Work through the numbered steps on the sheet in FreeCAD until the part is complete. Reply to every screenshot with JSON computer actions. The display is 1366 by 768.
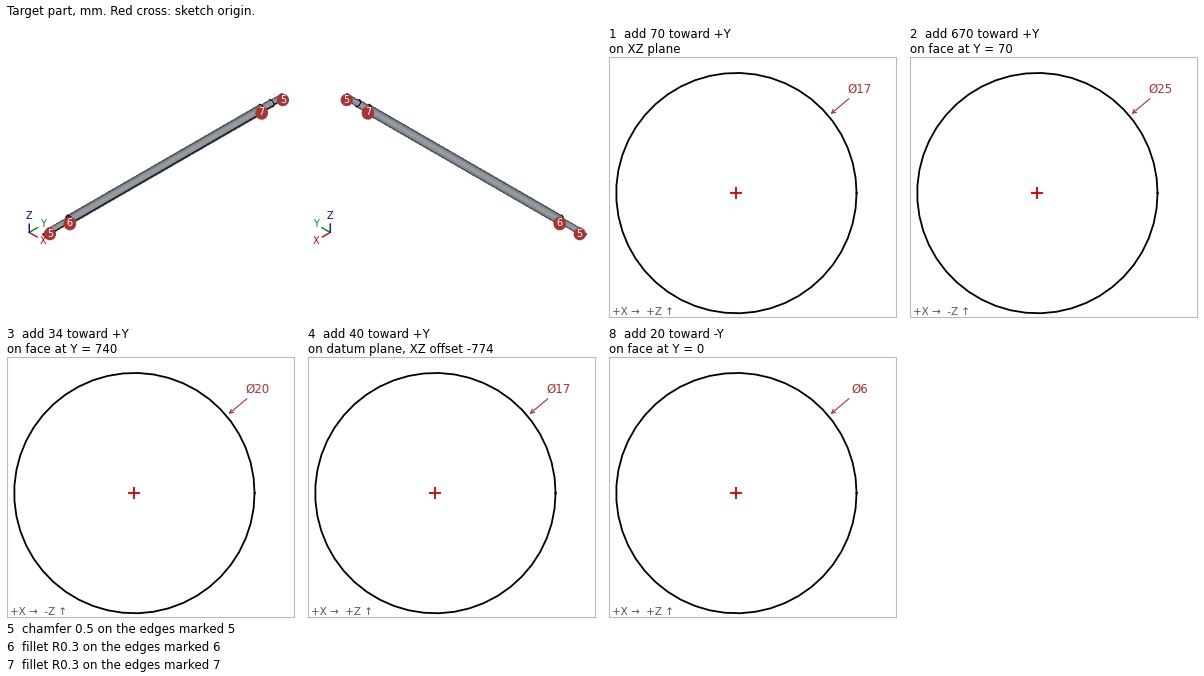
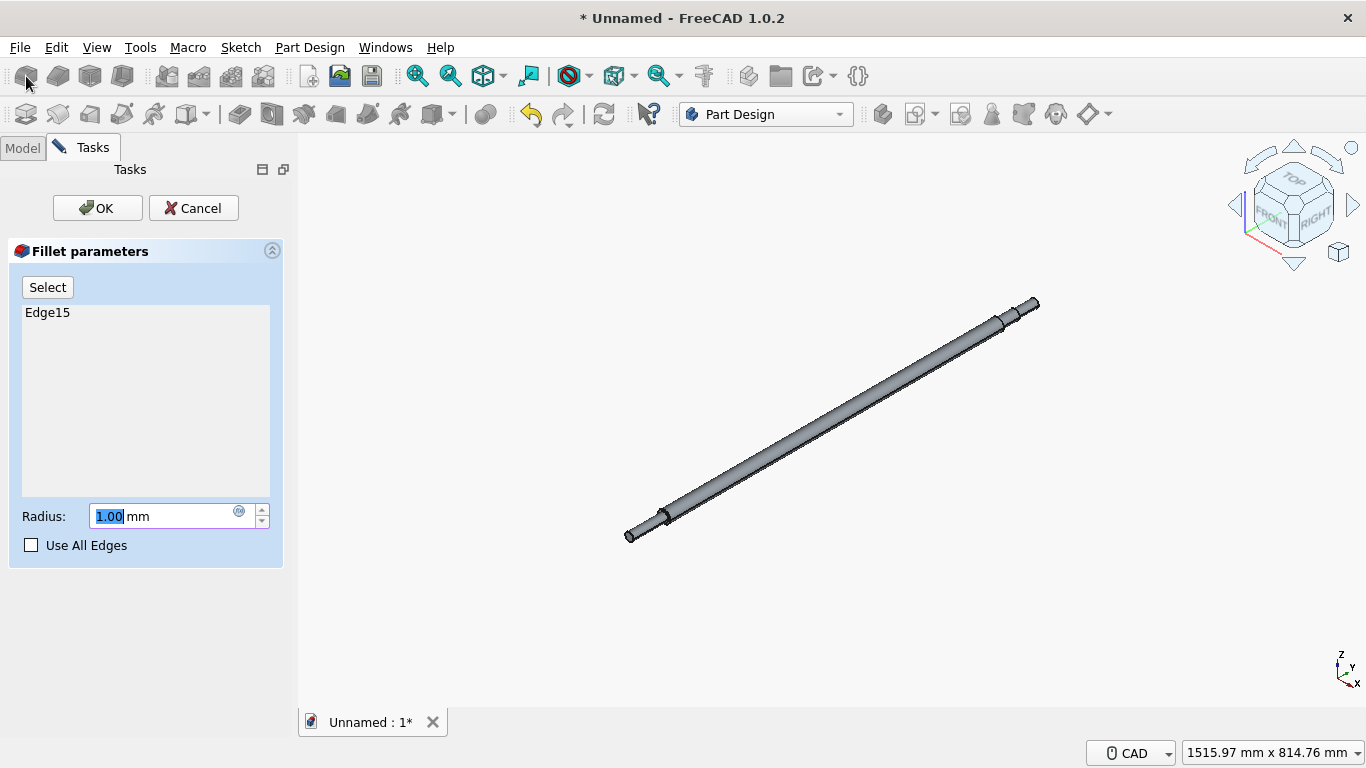
{"action": "type", "text": "0.3"}
{"action": "key", "text": "Tab"}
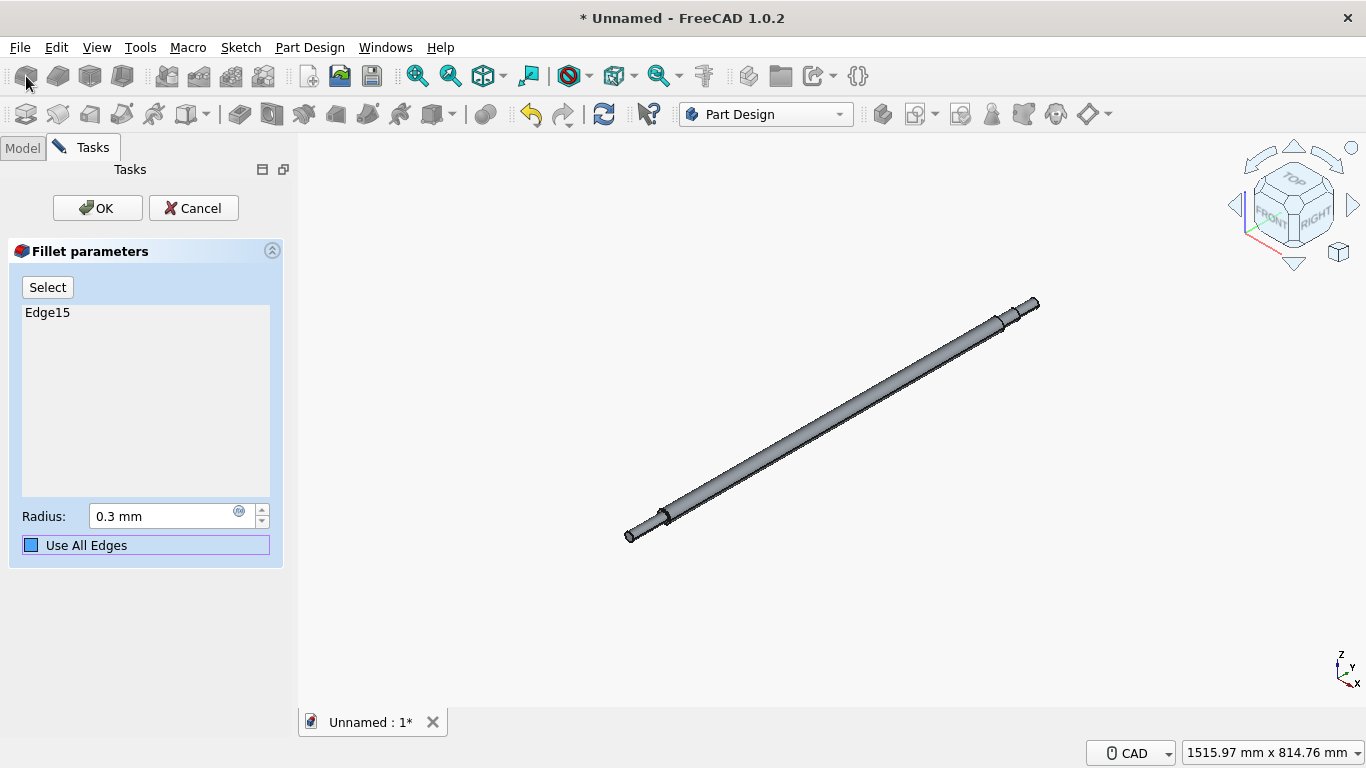
{"action": "left_click", "coordinate": [98, 208]}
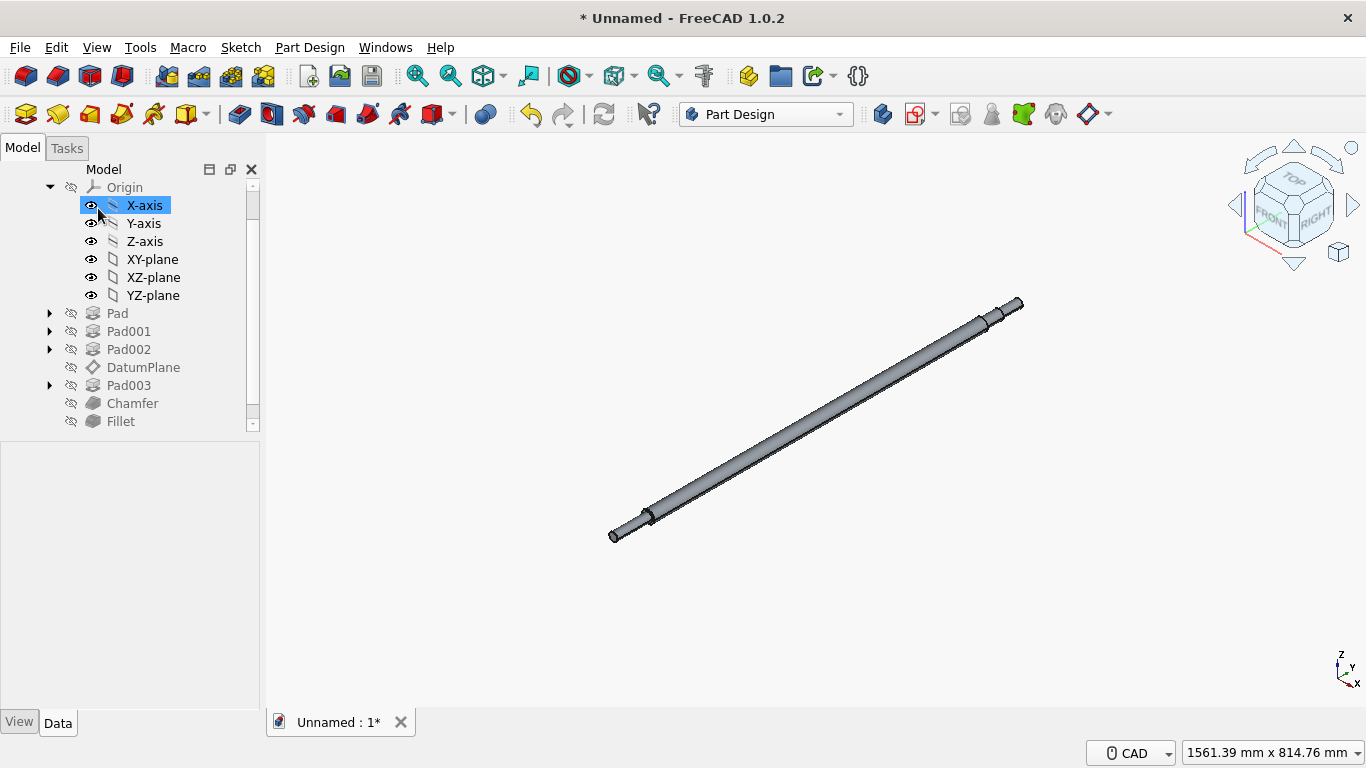
{"action": "left_click", "coordinate": [418, 76]}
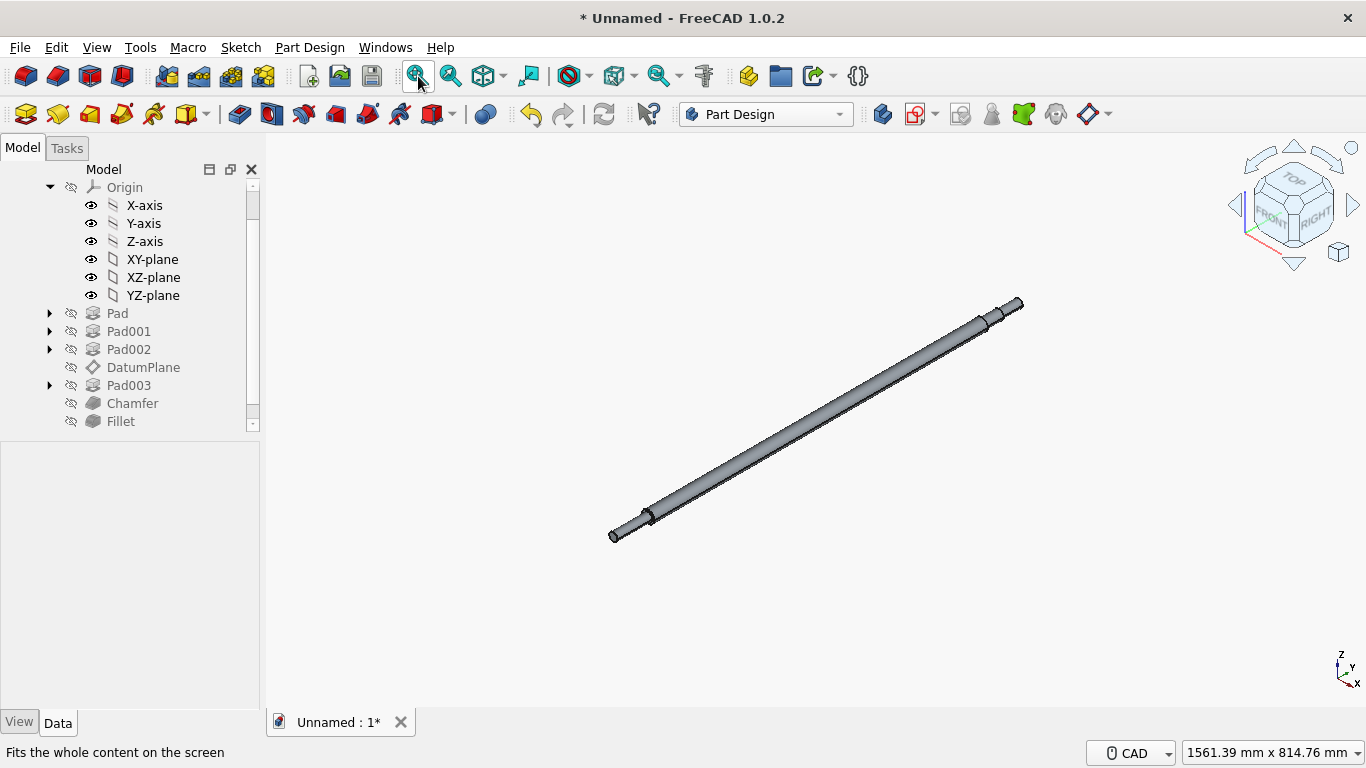
{"action": "scroll", "coordinate": [613, 536], "scroll_direction": "up", "scroll_amount": 4}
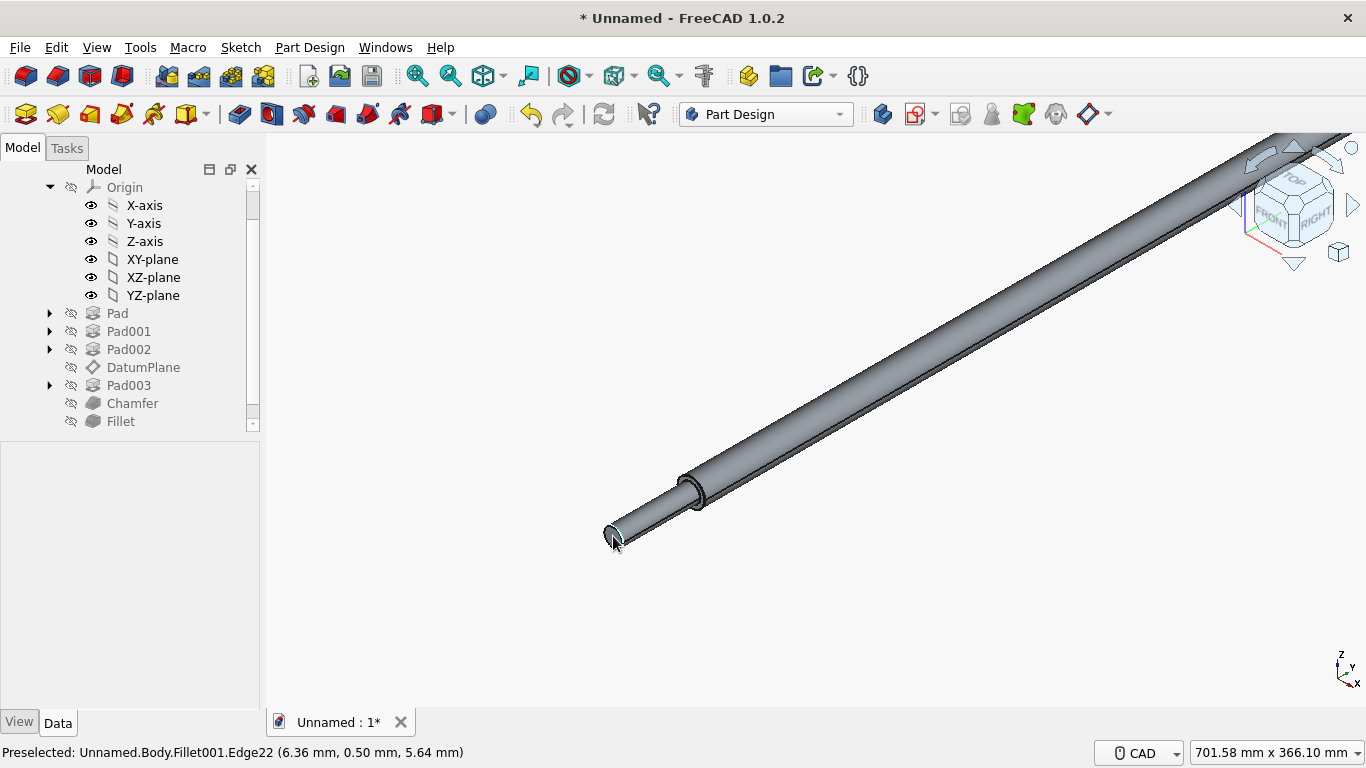
{"action": "left_click", "coordinate": [418, 76]}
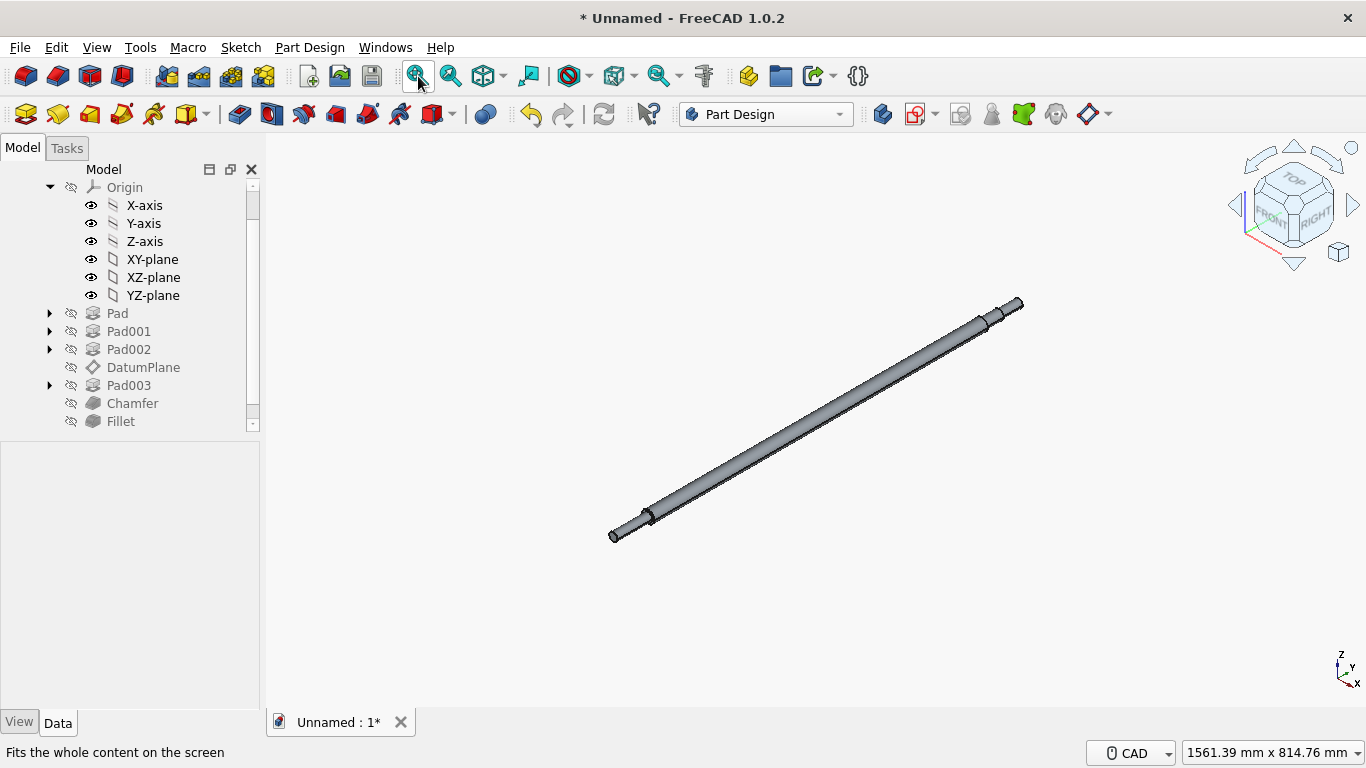
{"action": "key", "text": "1"}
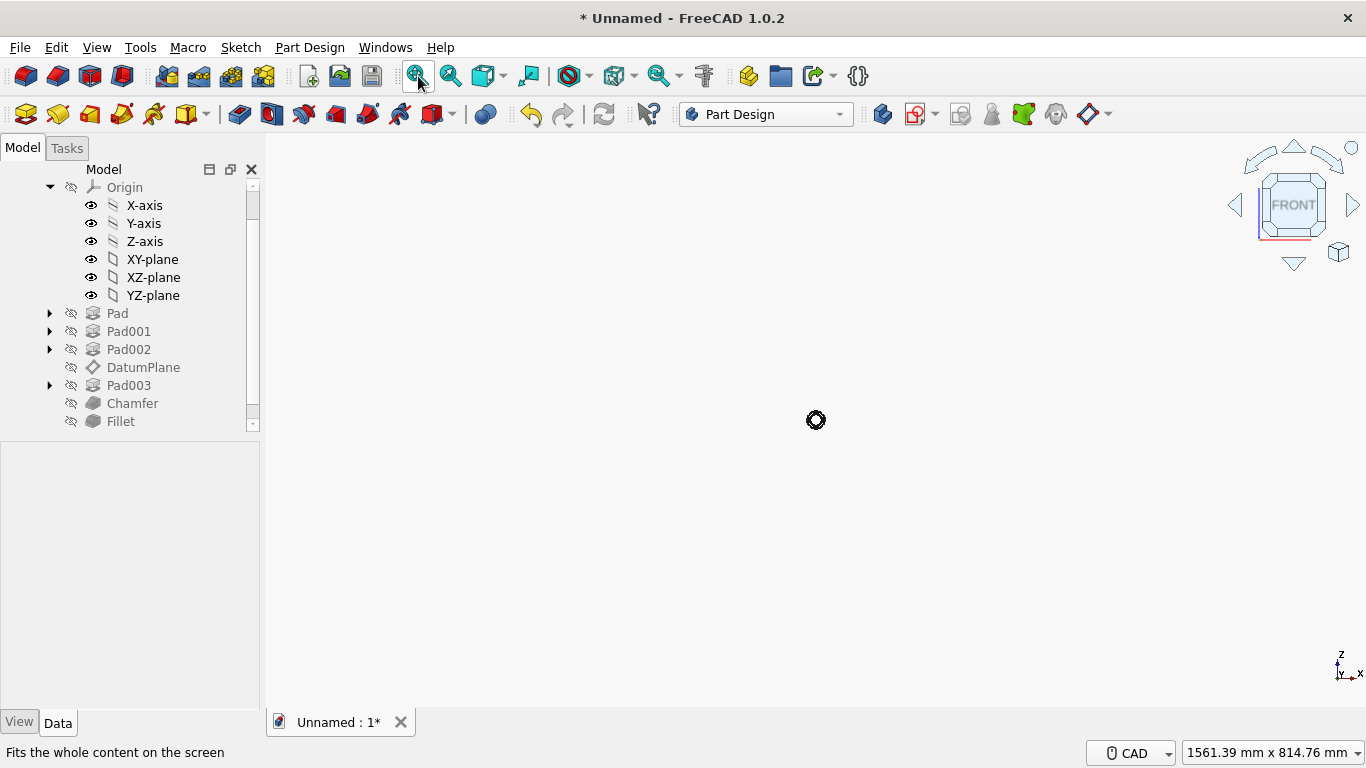
{"action": "key", "text": "v f"}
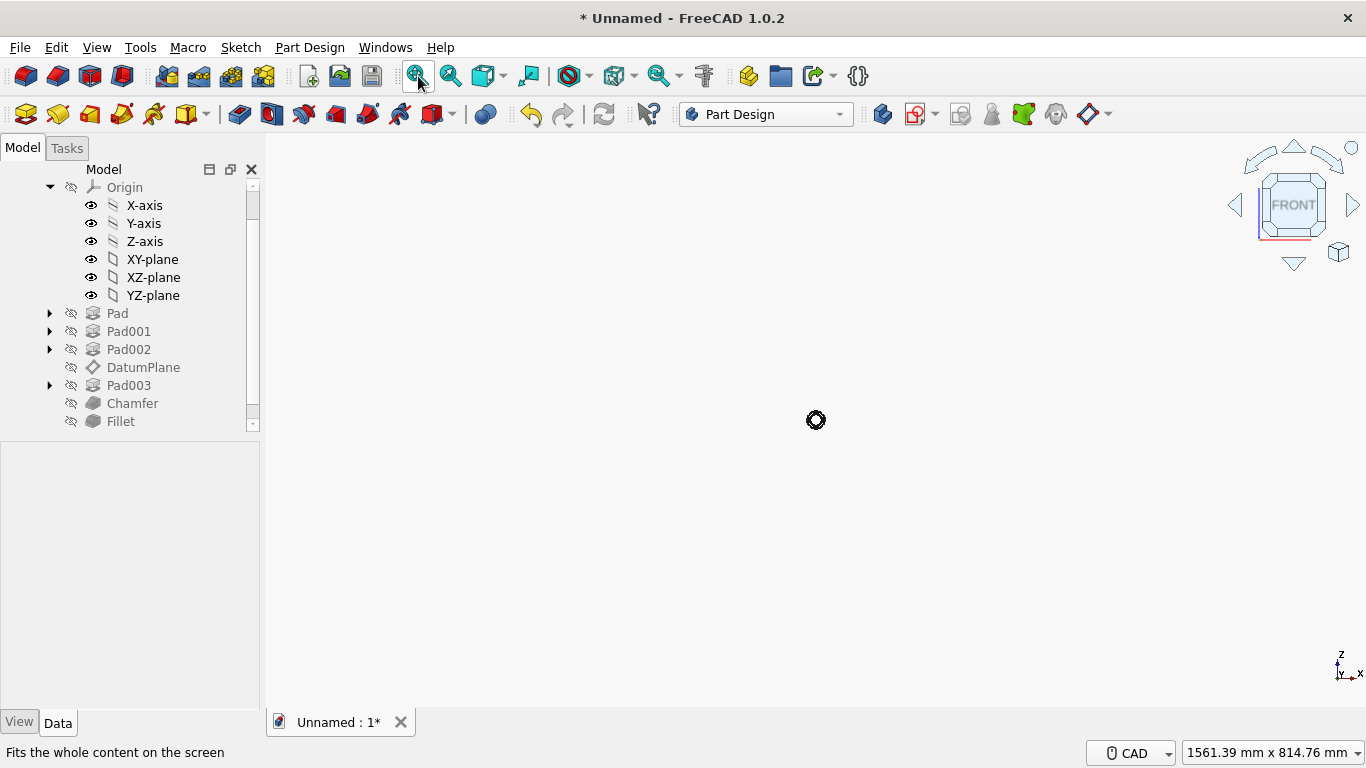
{"action": "scroll", "coordinate": [816, 419], "scroll_direction": "up", "scroll_amount": 4}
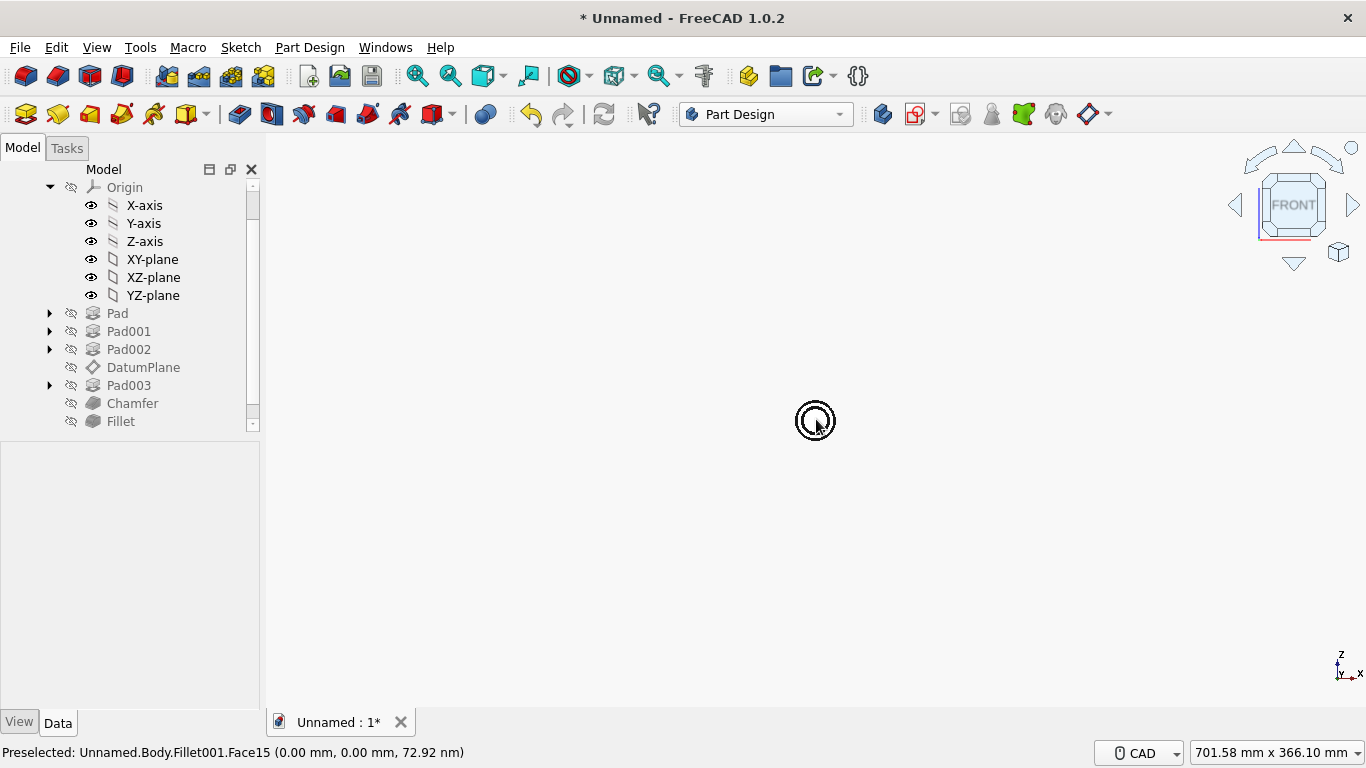
{"action": "left_click", "coordinate": [815, 420]}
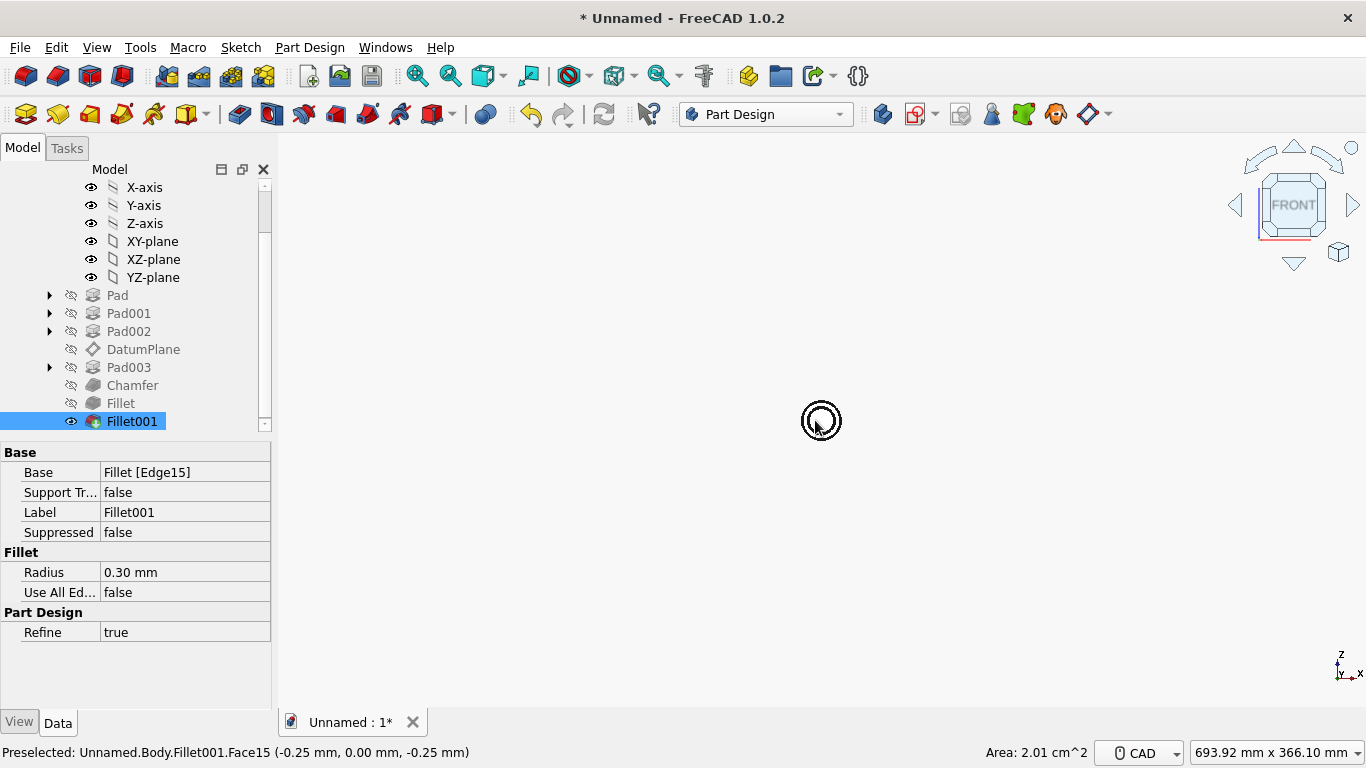
{"action": "left_click", "coordinate": [916, 114]}